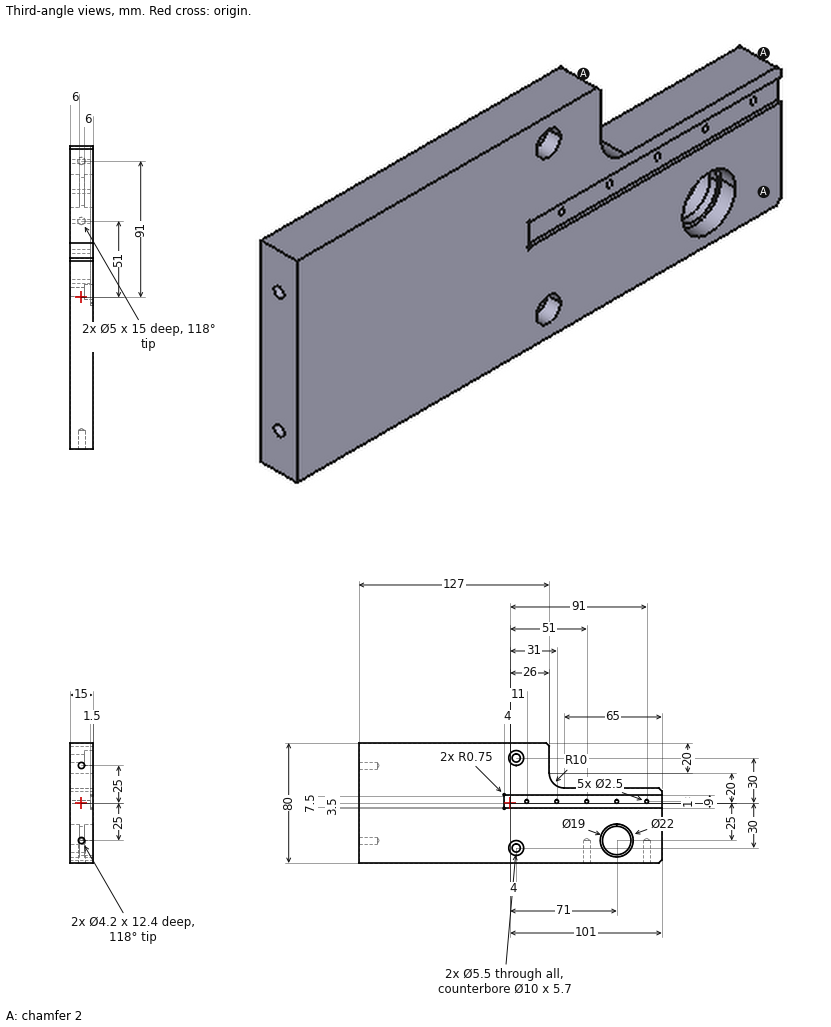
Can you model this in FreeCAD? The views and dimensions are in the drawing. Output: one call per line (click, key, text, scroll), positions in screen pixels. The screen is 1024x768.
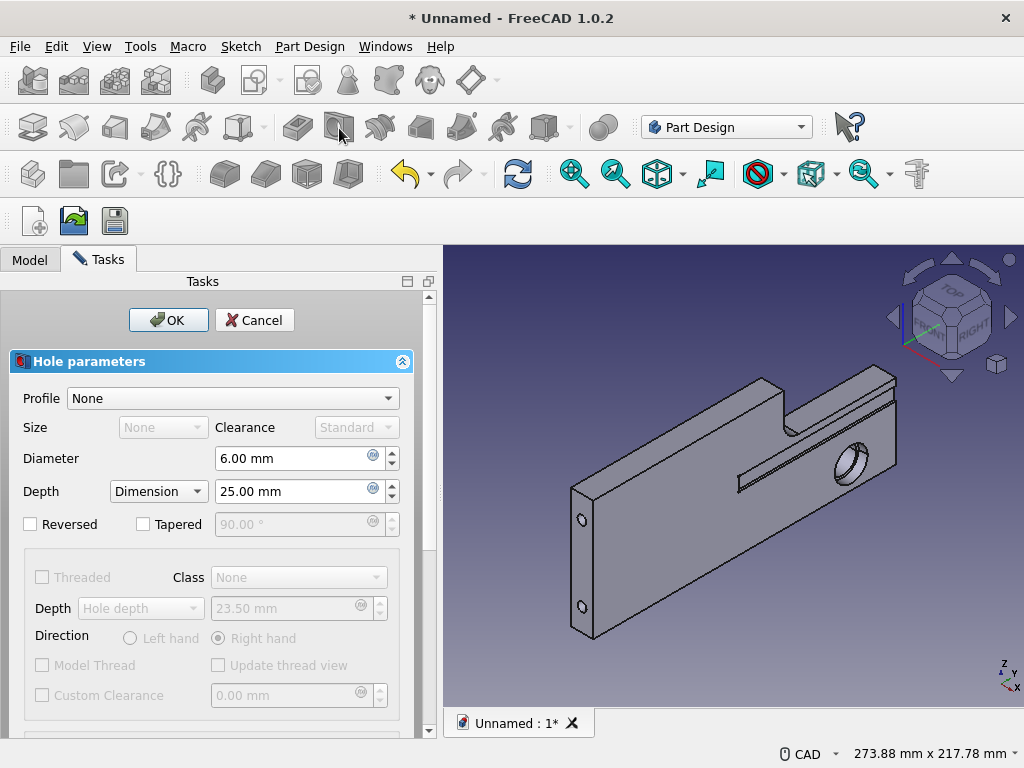
triple_click(300, 458)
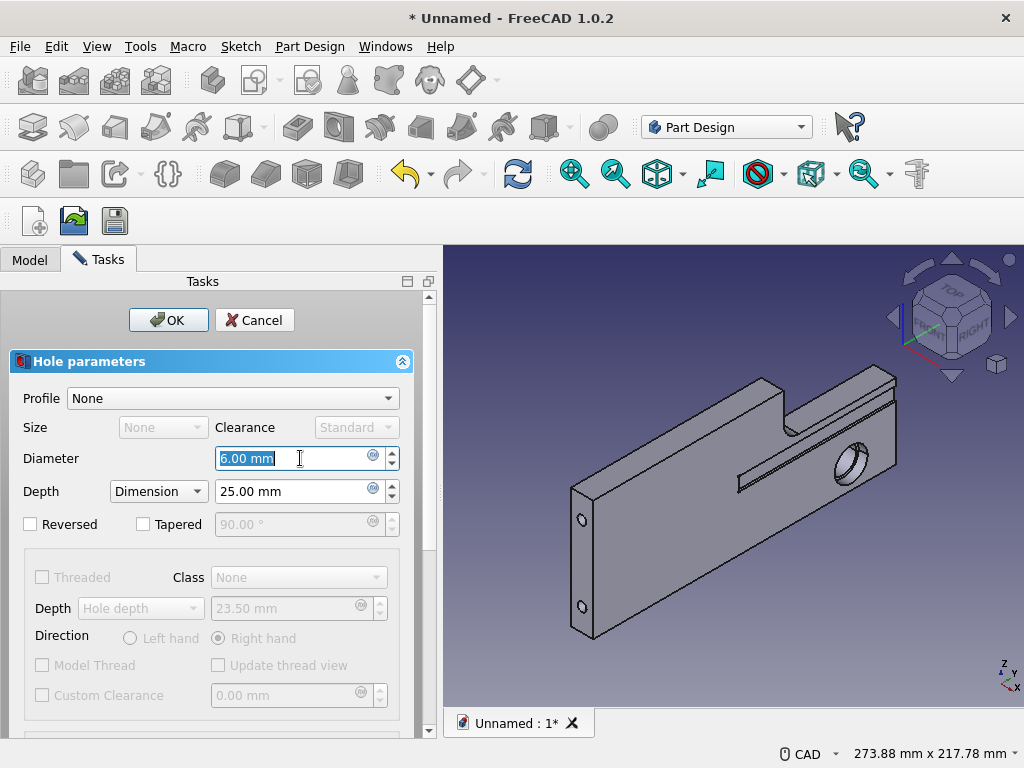
text(4.2)
key(Tab)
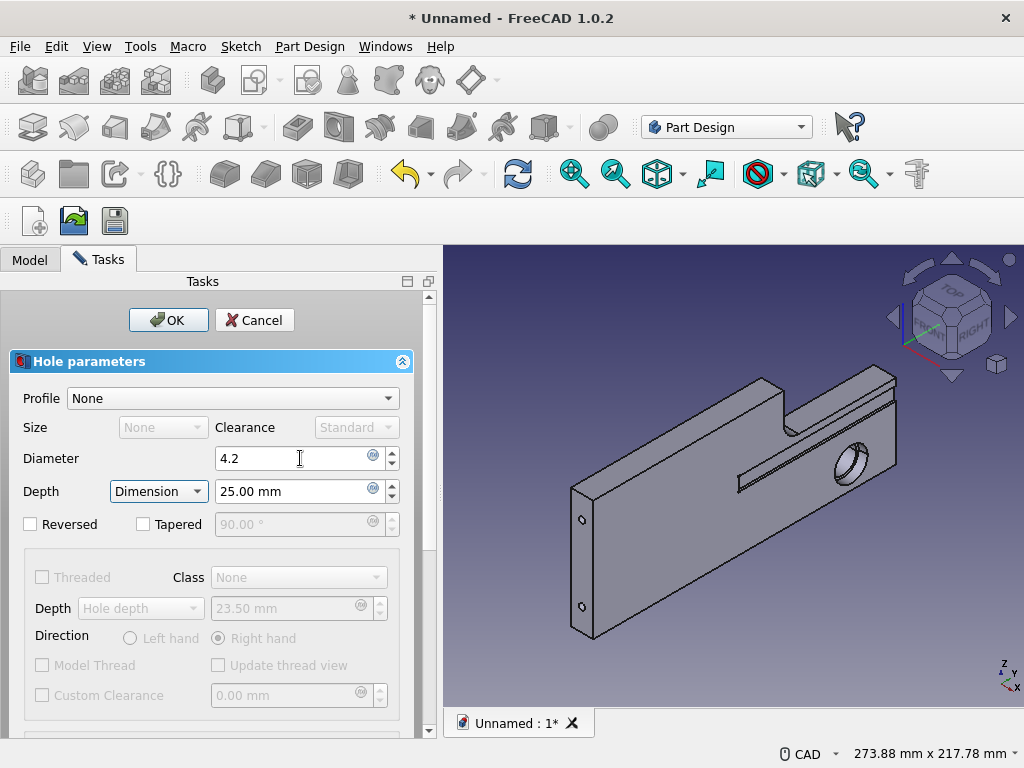
triple_click(300, 492)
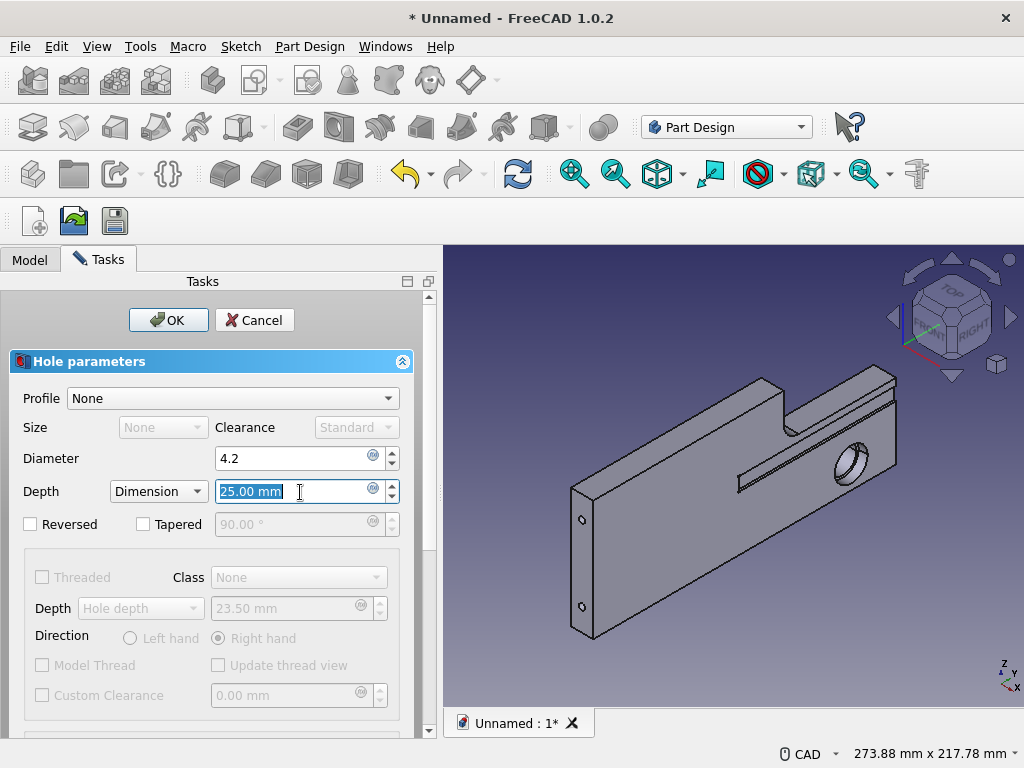
text(12.4)
key(Tab)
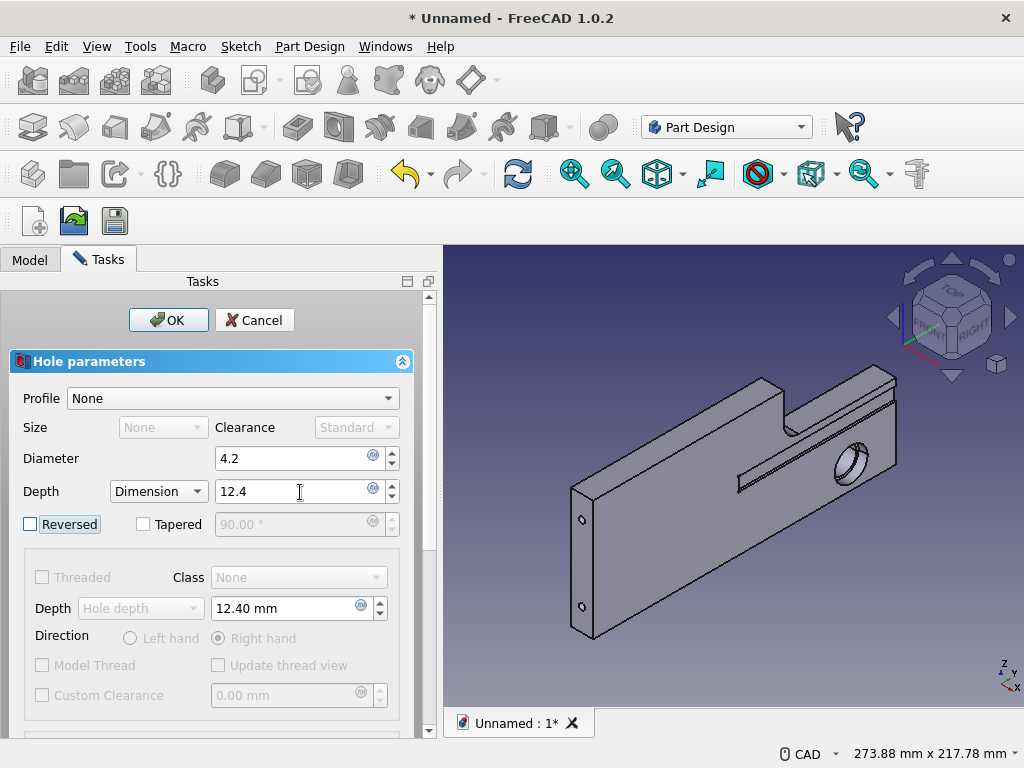
click(169, 320)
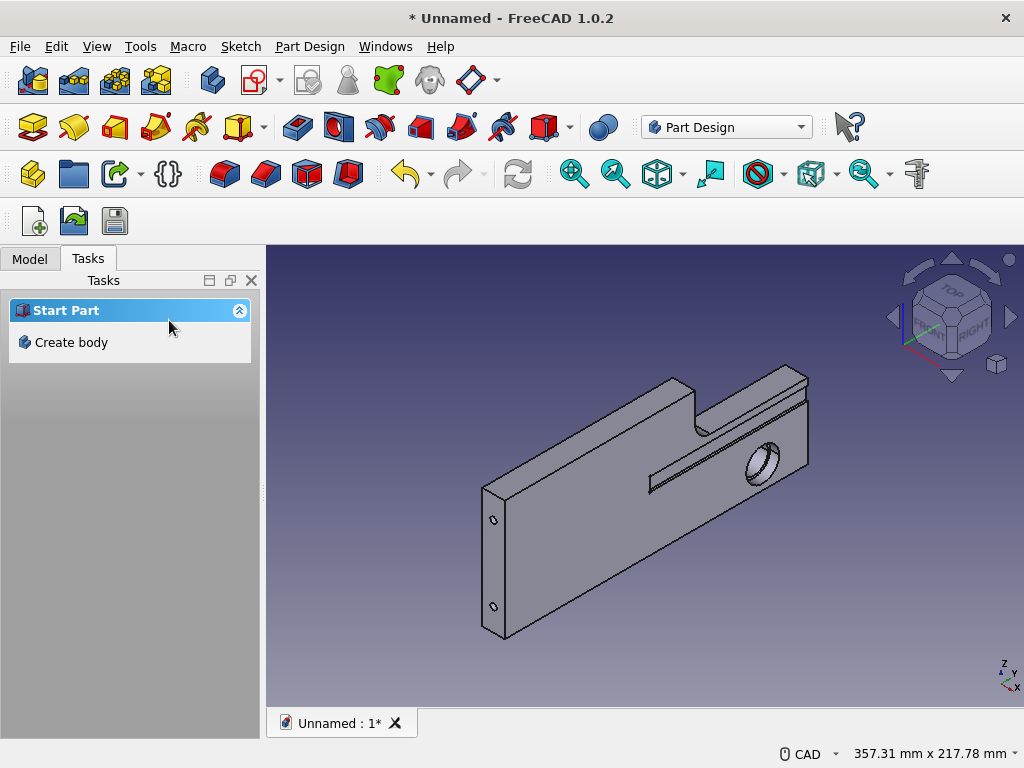
click(570, 531)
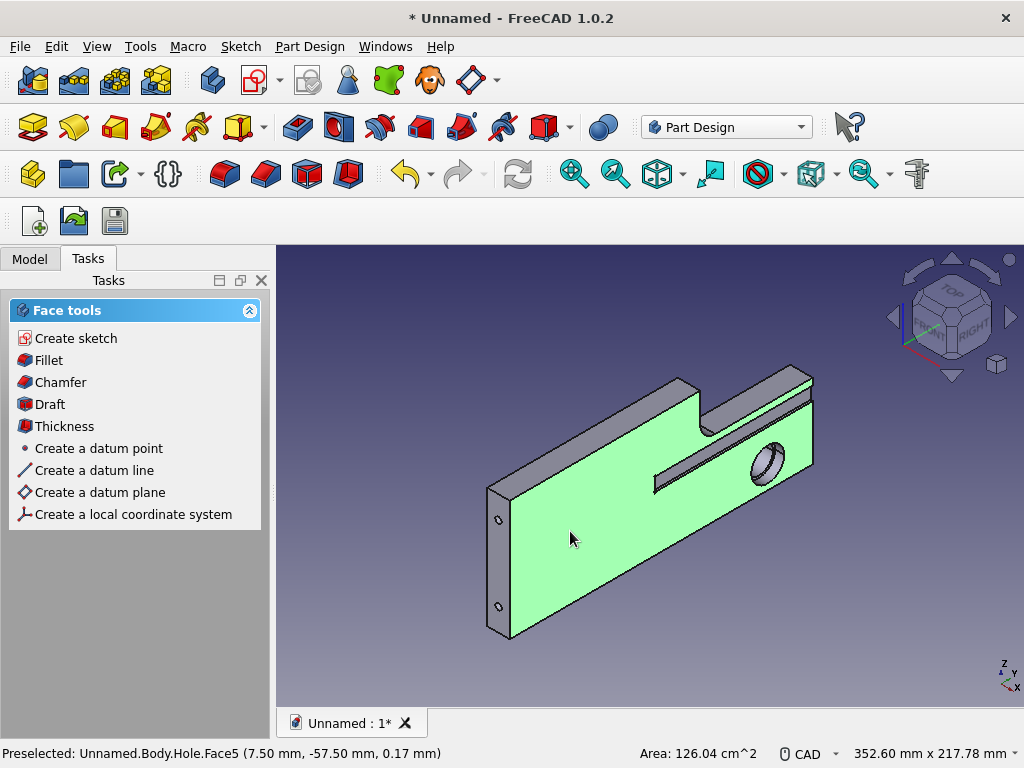
click(254, 80)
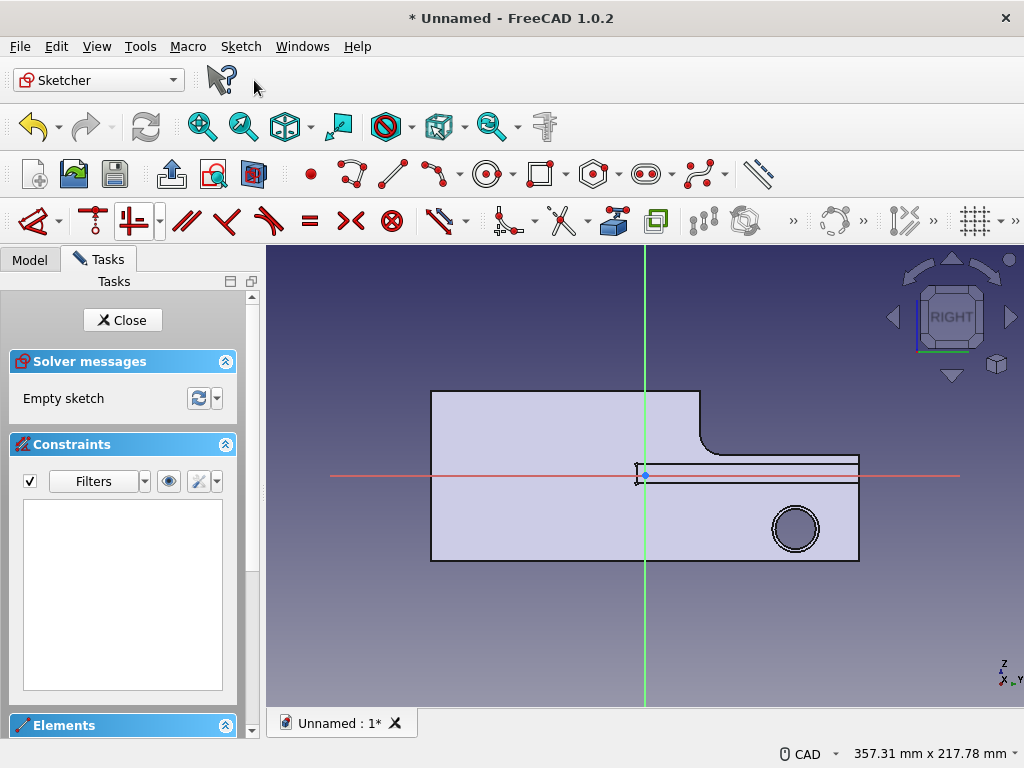
scroll(714, 476, up, 4)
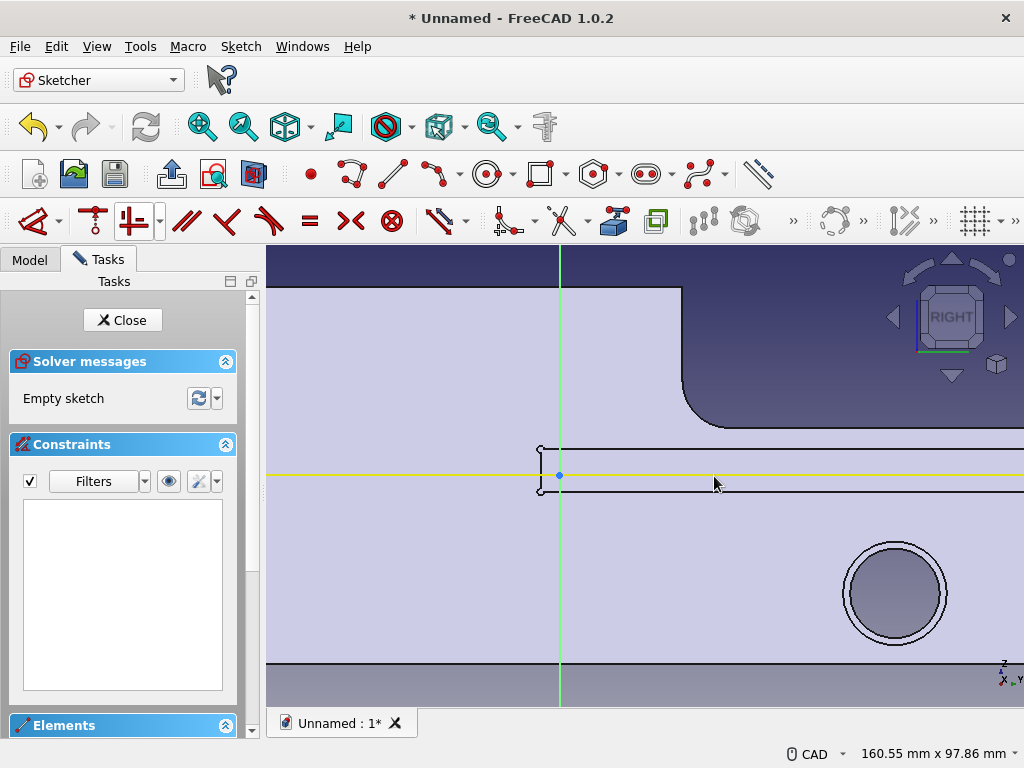
click(486, 174)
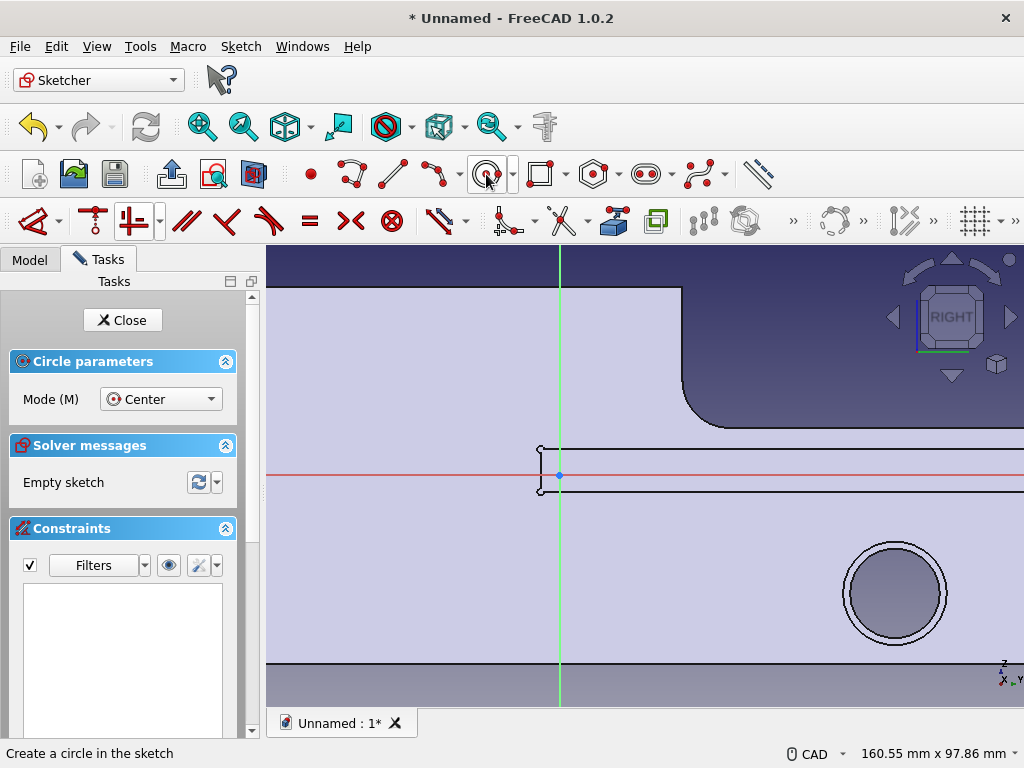
scroll(579, 617, up, 3)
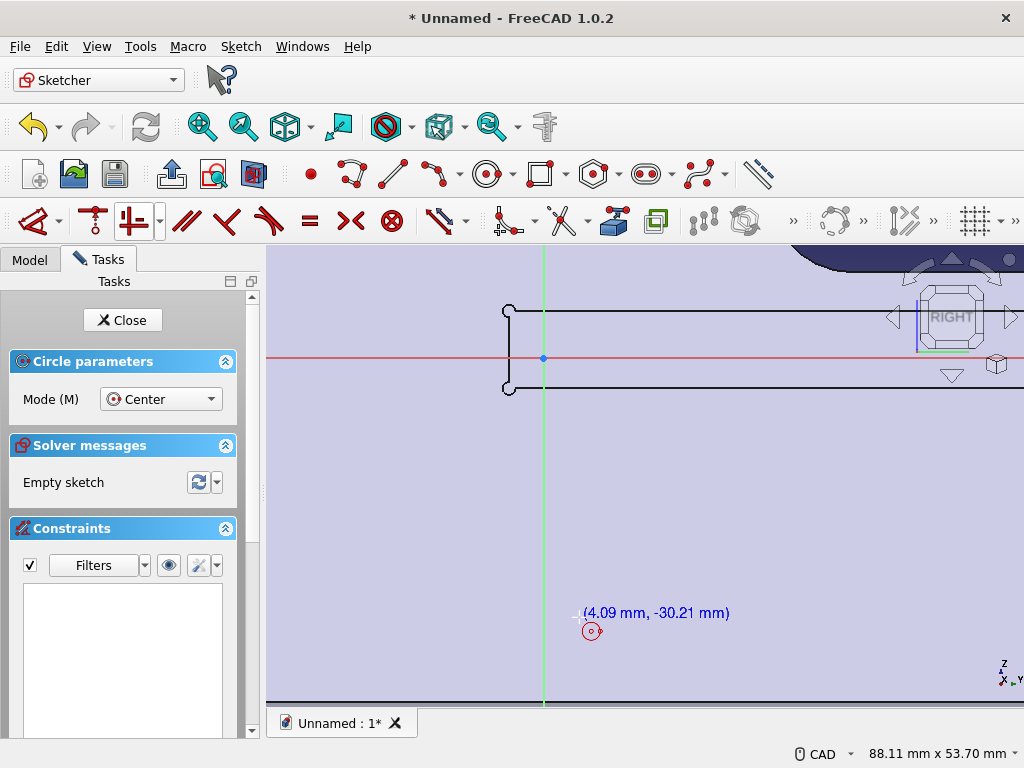
click(578, 616)
click(595, 600)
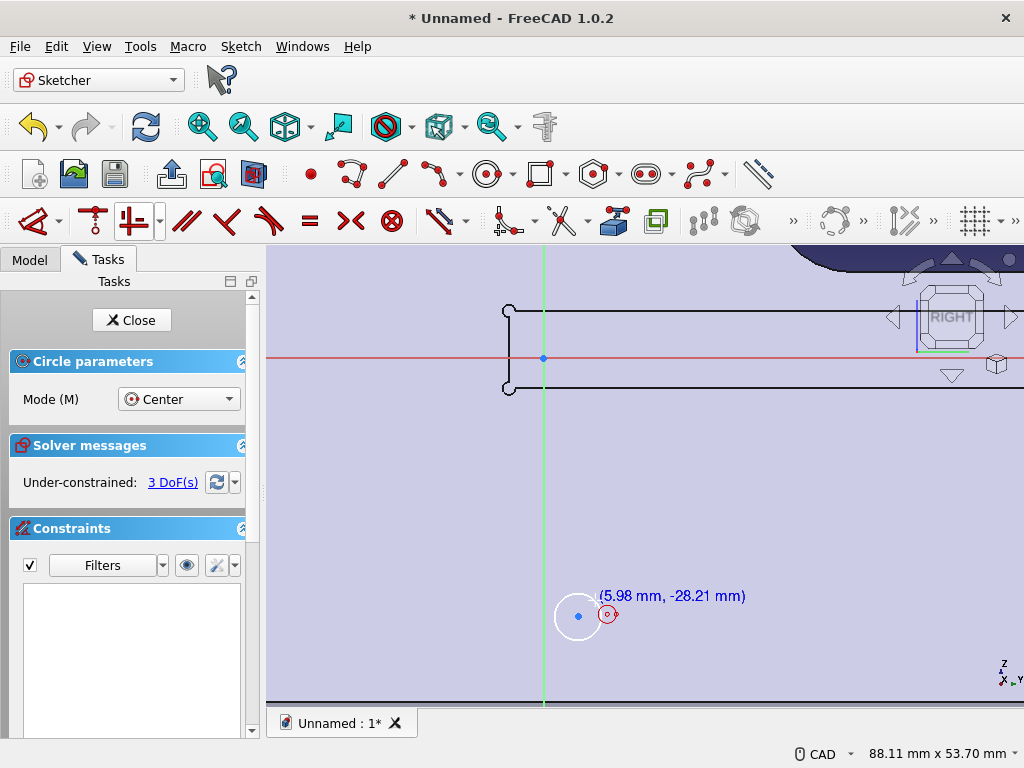
scroll(581, 619, down, 3)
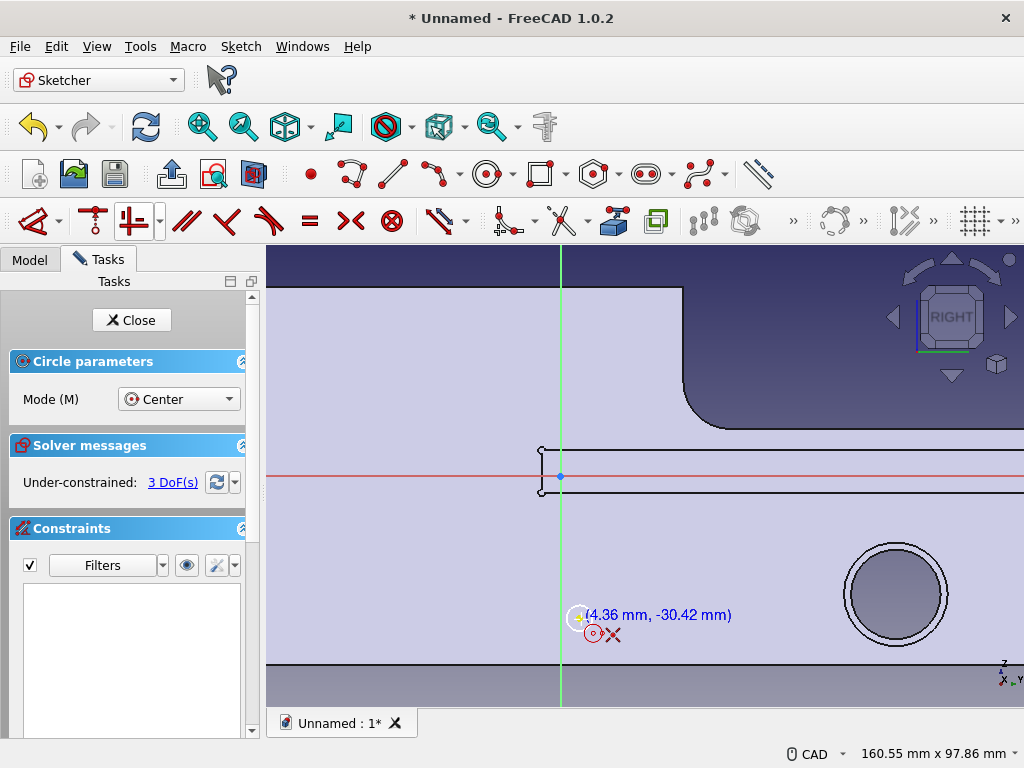
scroll(580, 335, up, 3)